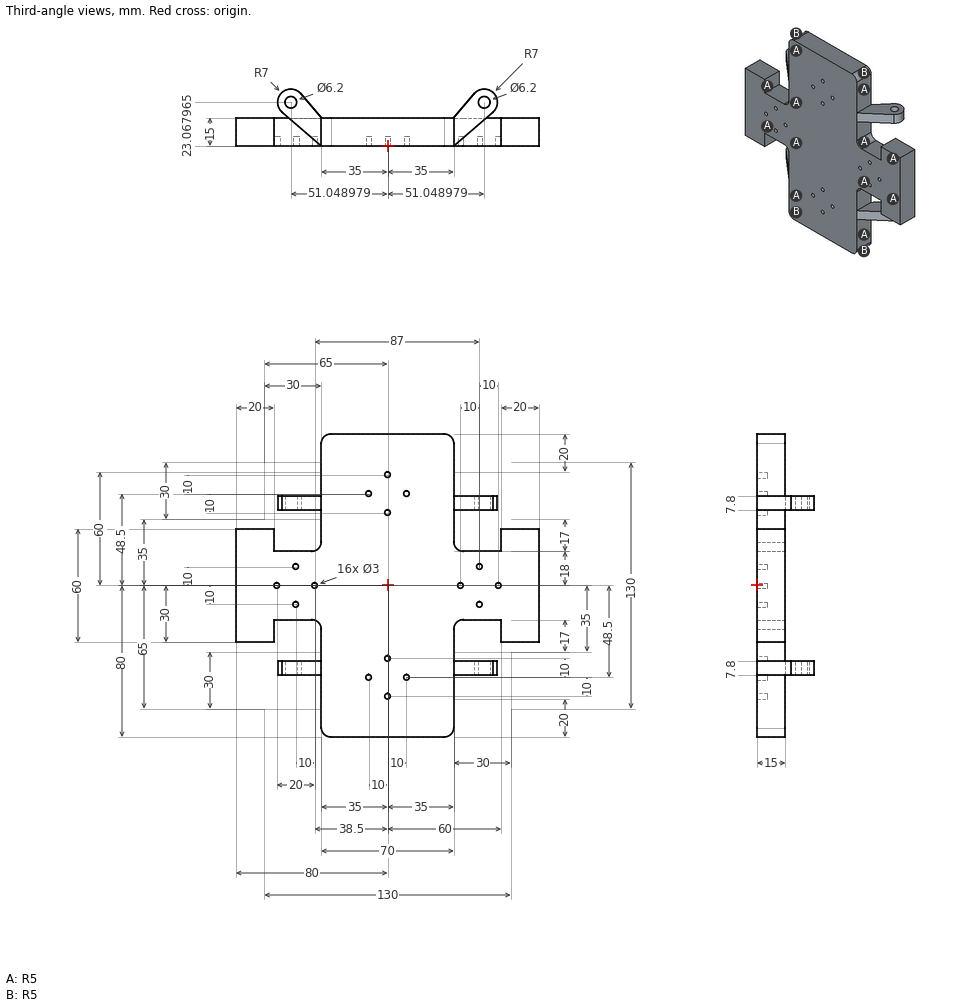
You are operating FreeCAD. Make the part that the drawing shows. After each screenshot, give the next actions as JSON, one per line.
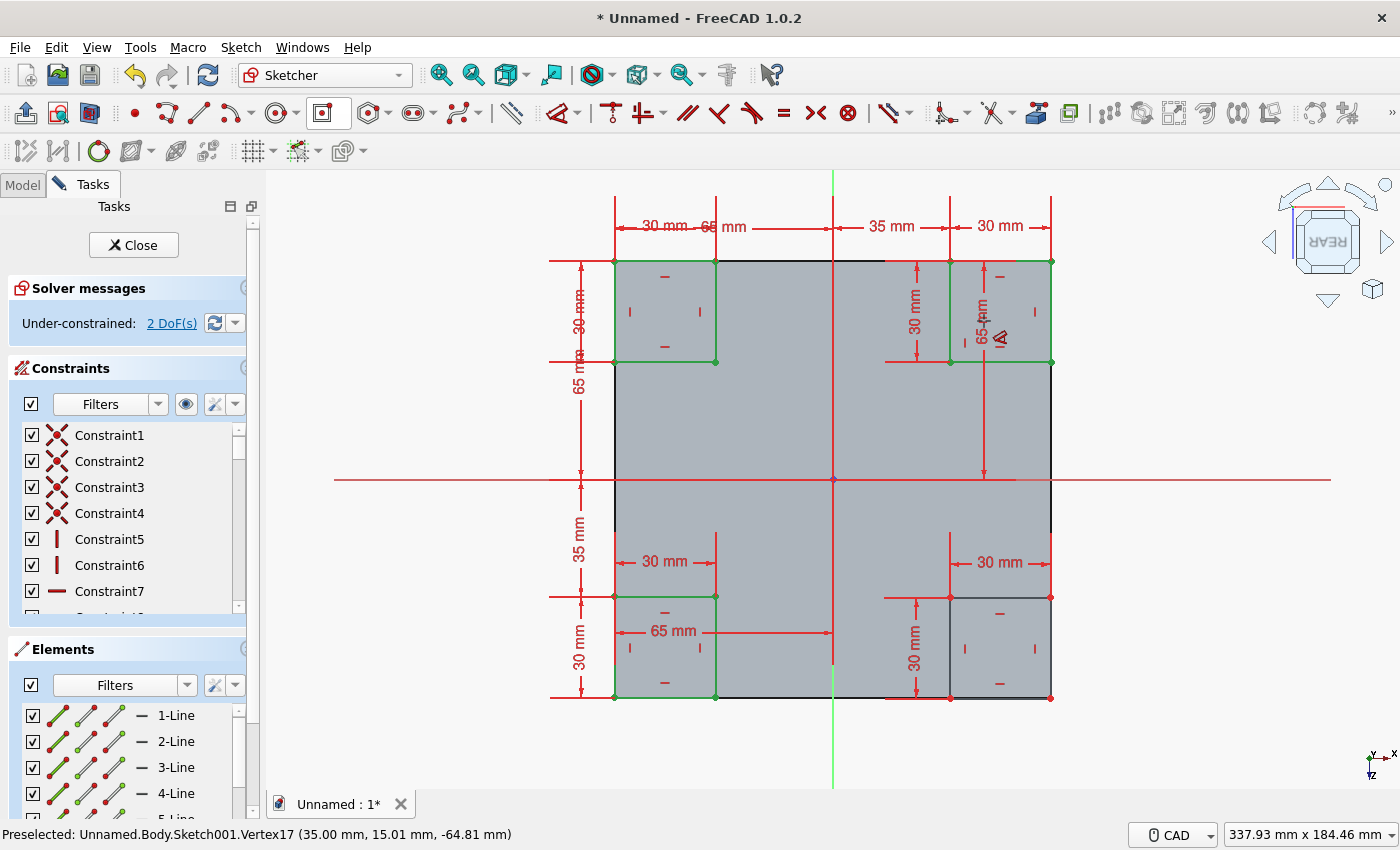
{"action": "left_click", "coordinate": [950, 598]}
{"action": "left_click", "coordinate": [892, 632]}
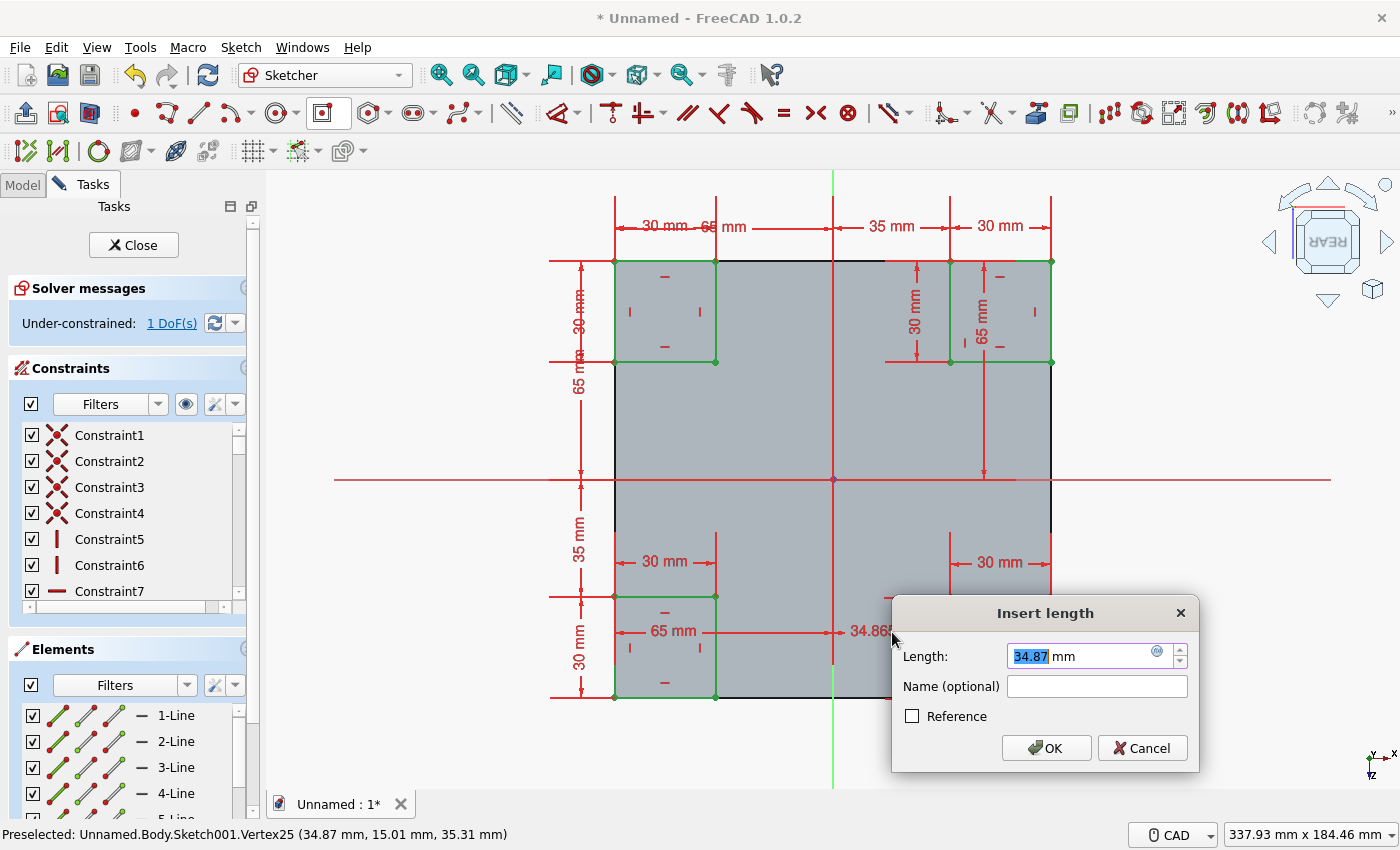
{"action": "type", "text": "35"}
{"action": "key", "text": "Return"}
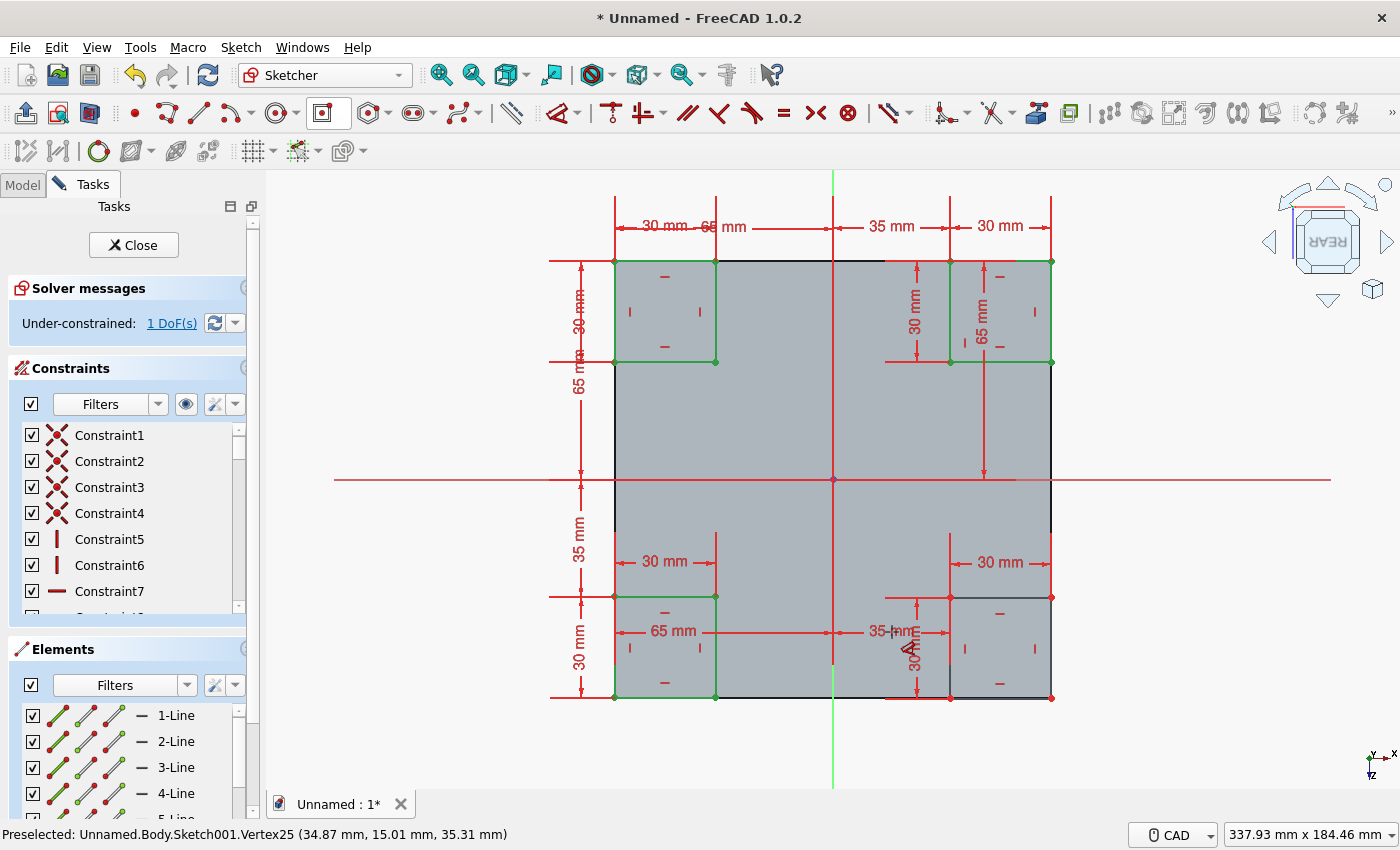
{"action": "left_click", "coordinate": [950, 598]}
{"action": "left_click", "coordinate": [984, 539]}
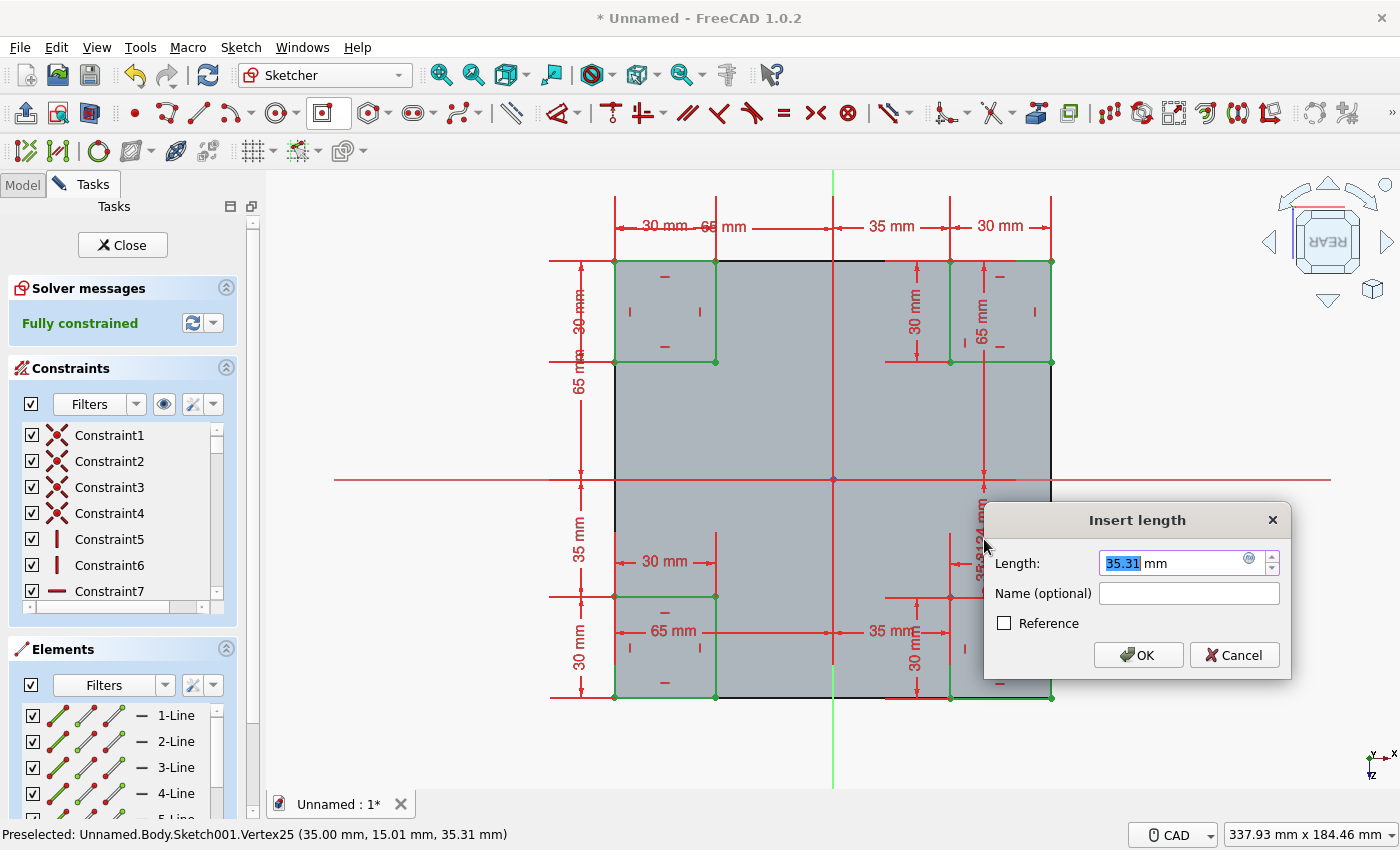
{"action": "type", "text": "35"}
{"action": "key", "text": "Return"}
{"action": "key", "text": "Escape"}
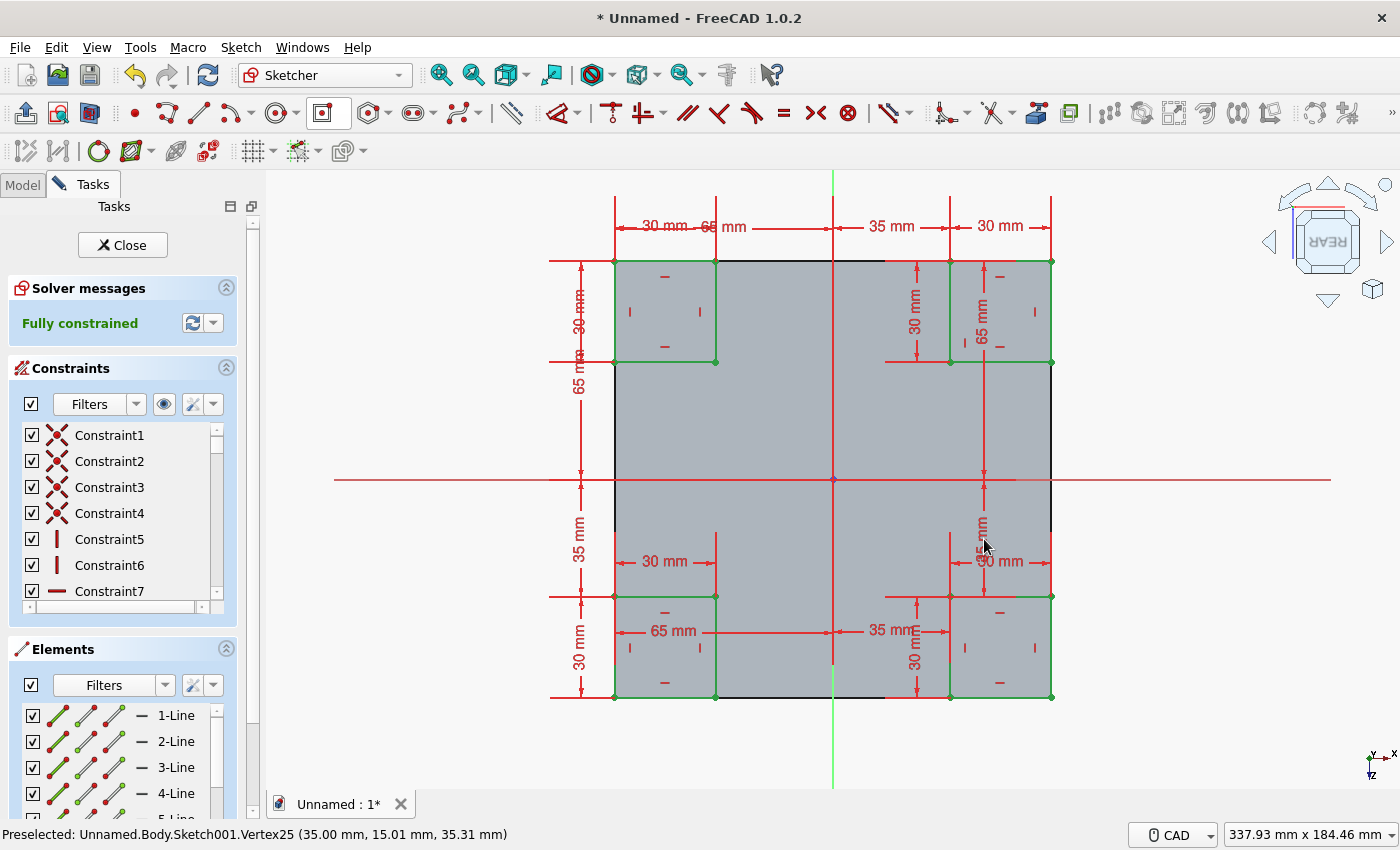
{"action": "left_click", "coordinate": [123, 245]}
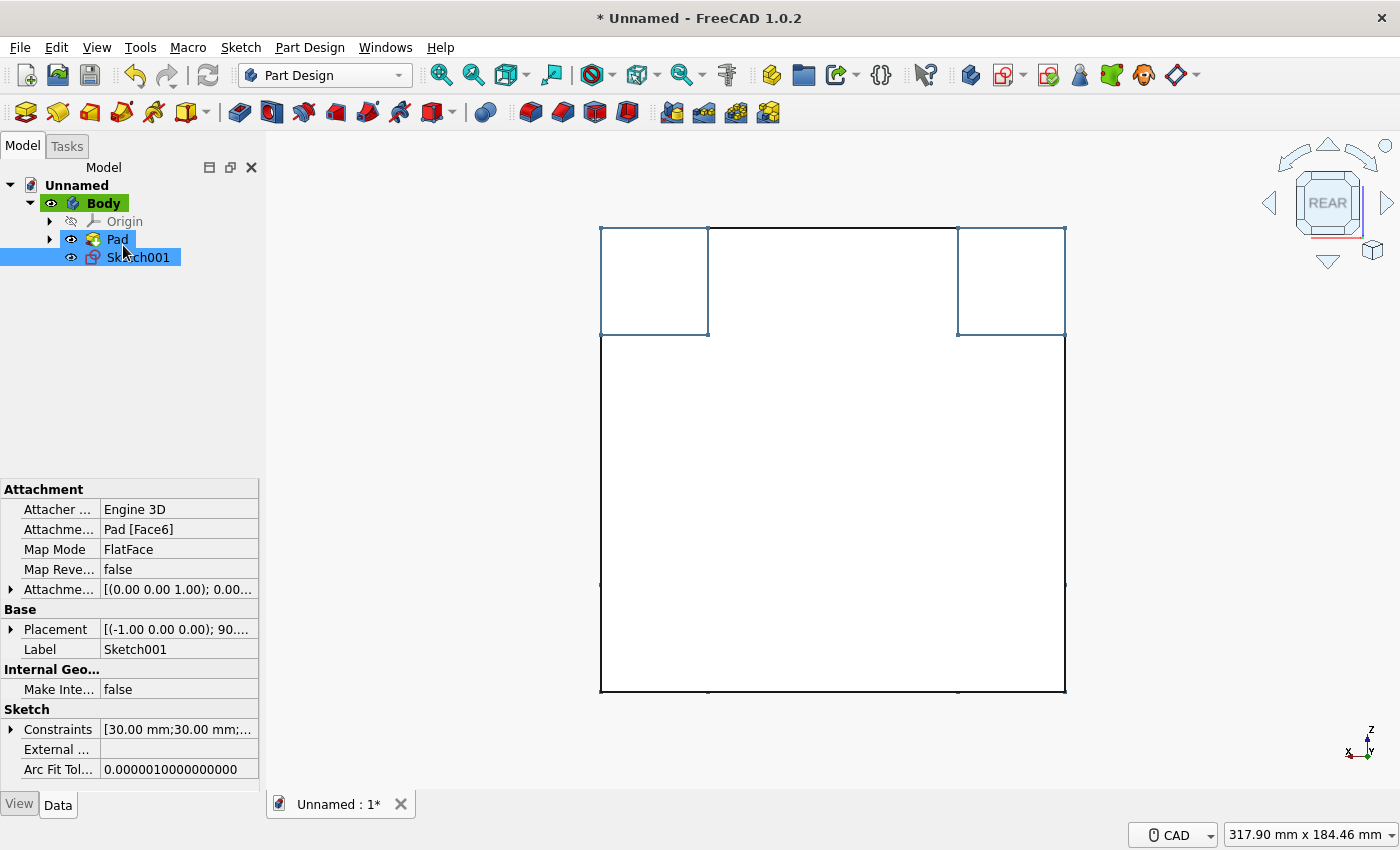
{"action": "left_click", "coordinate": [240, 112]}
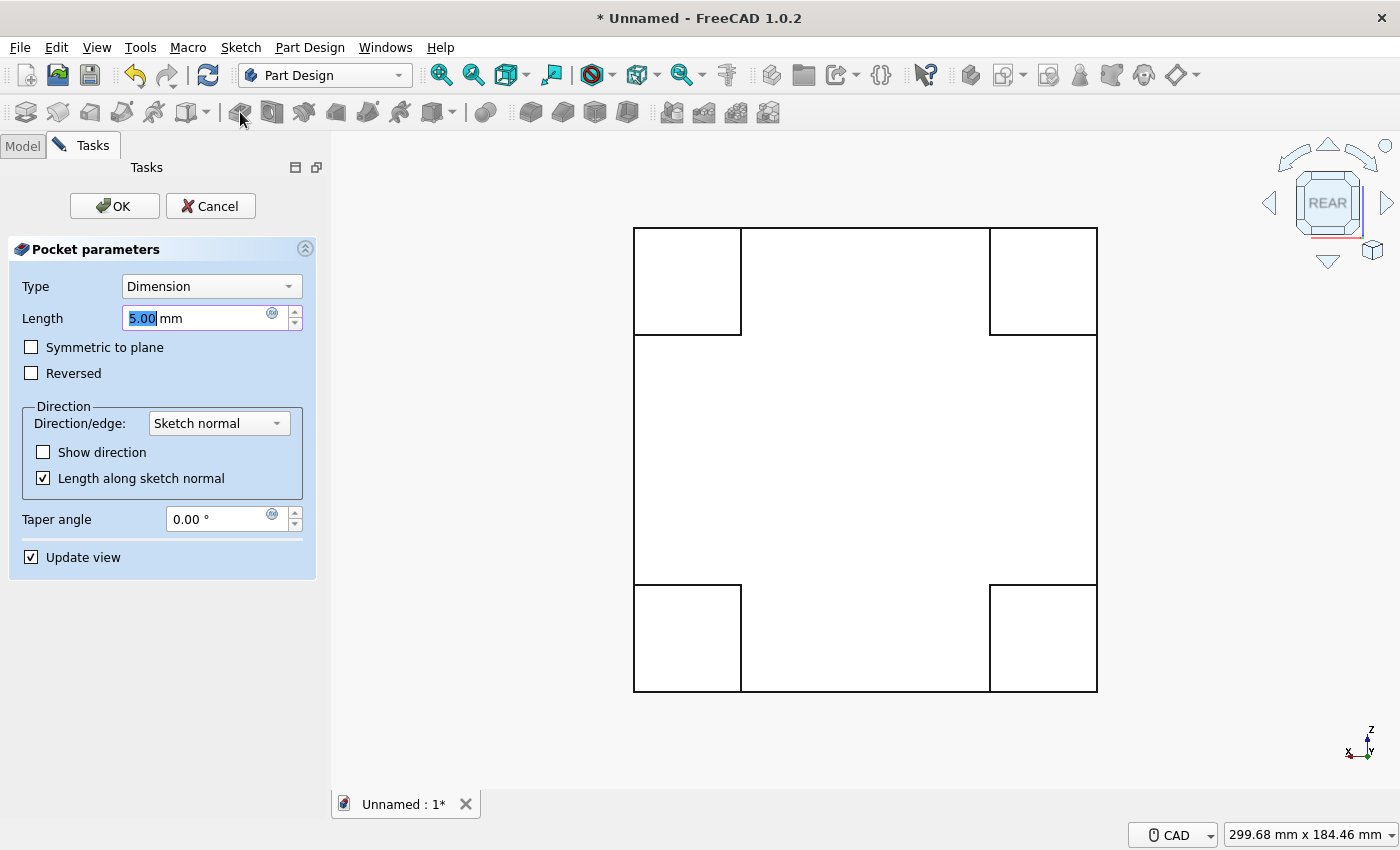
{"action": "left_click", "coordinate": [212, 286]}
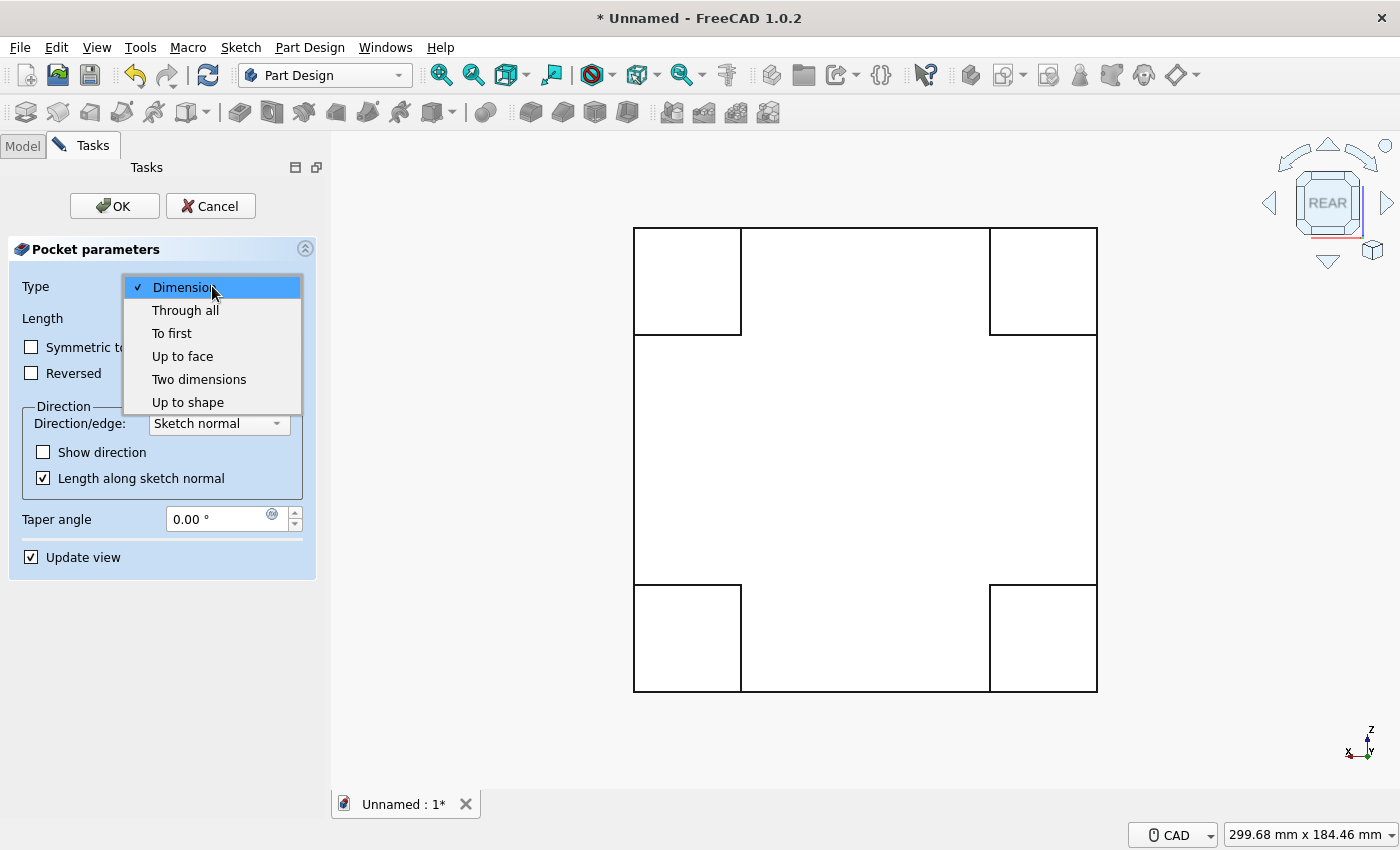
{"action": "left_click", "coordinate": [212, 310]}